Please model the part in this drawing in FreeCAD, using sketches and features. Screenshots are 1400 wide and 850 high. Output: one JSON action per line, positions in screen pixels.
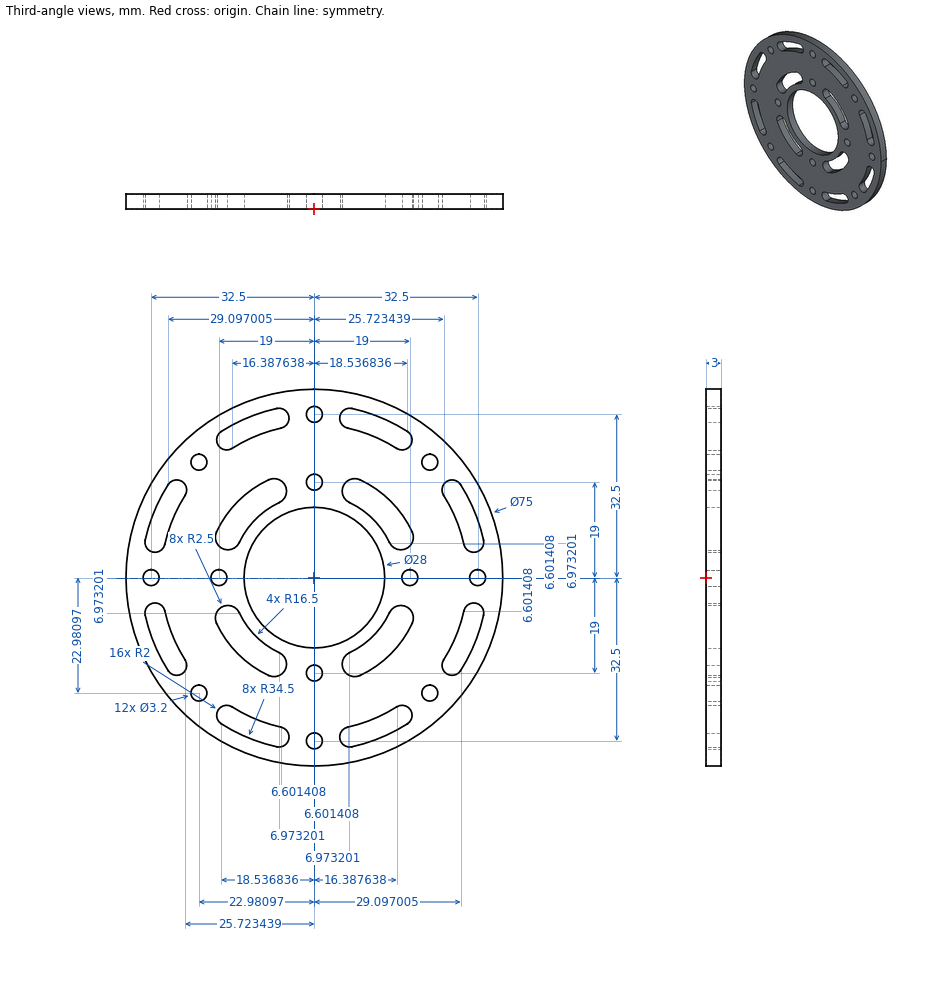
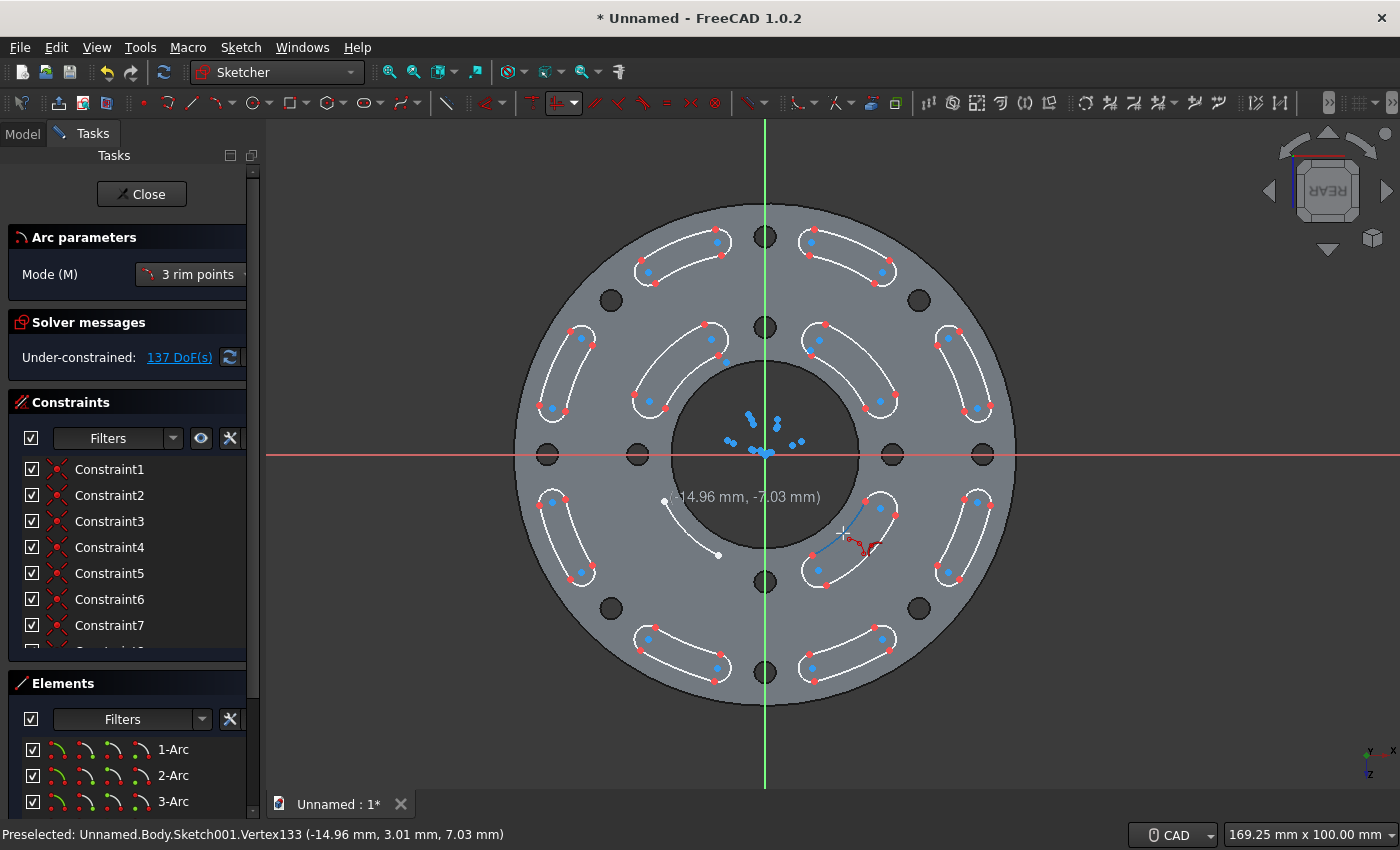
{"action": "left_click", "coordinate": [635, 516]}
{"action": "left_click", "coordinate": [643, 493]}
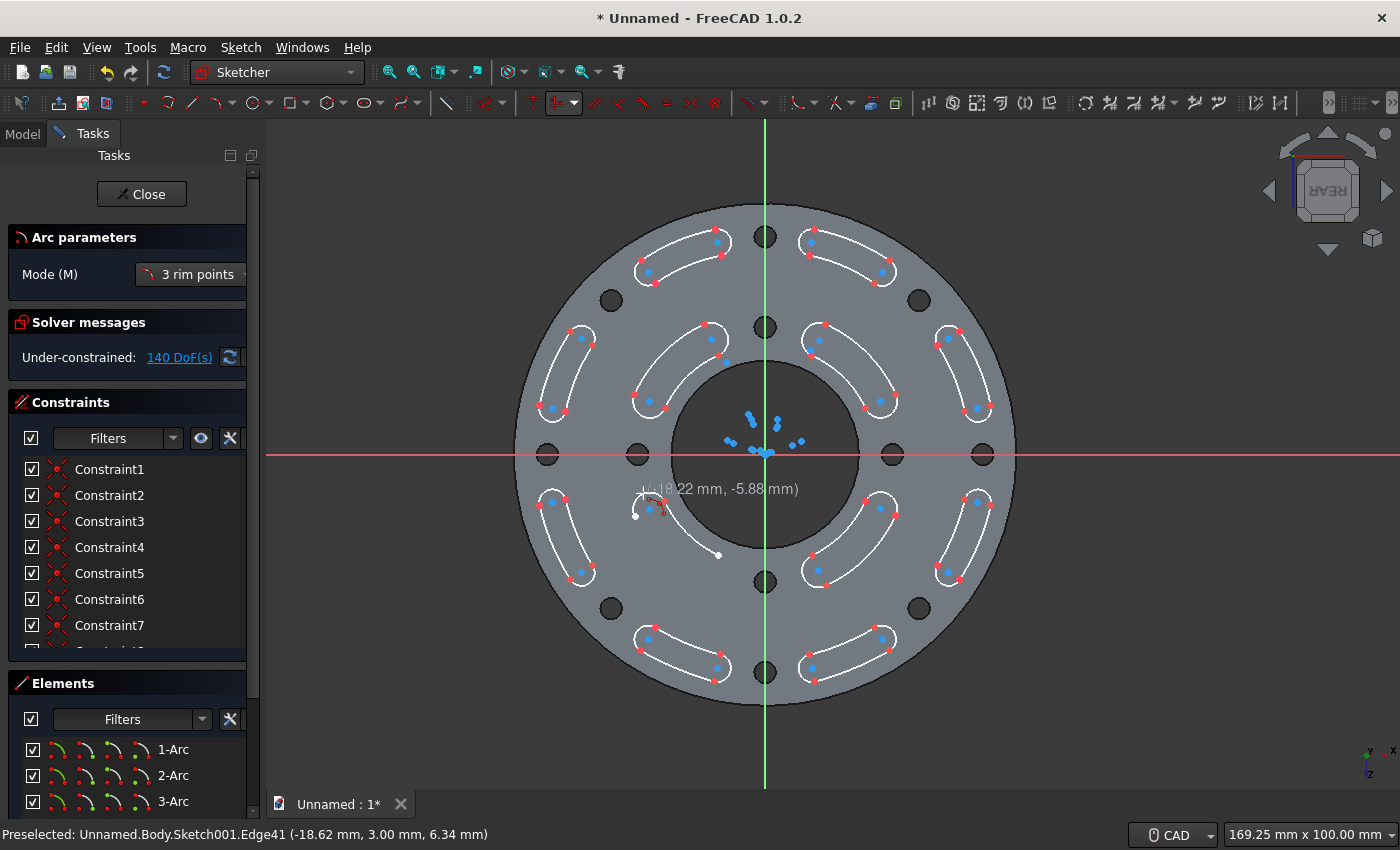
{"action": "left_click", "coordinate": [635, 517]}
{"action": "left_click", "coordinate": [704, 585]}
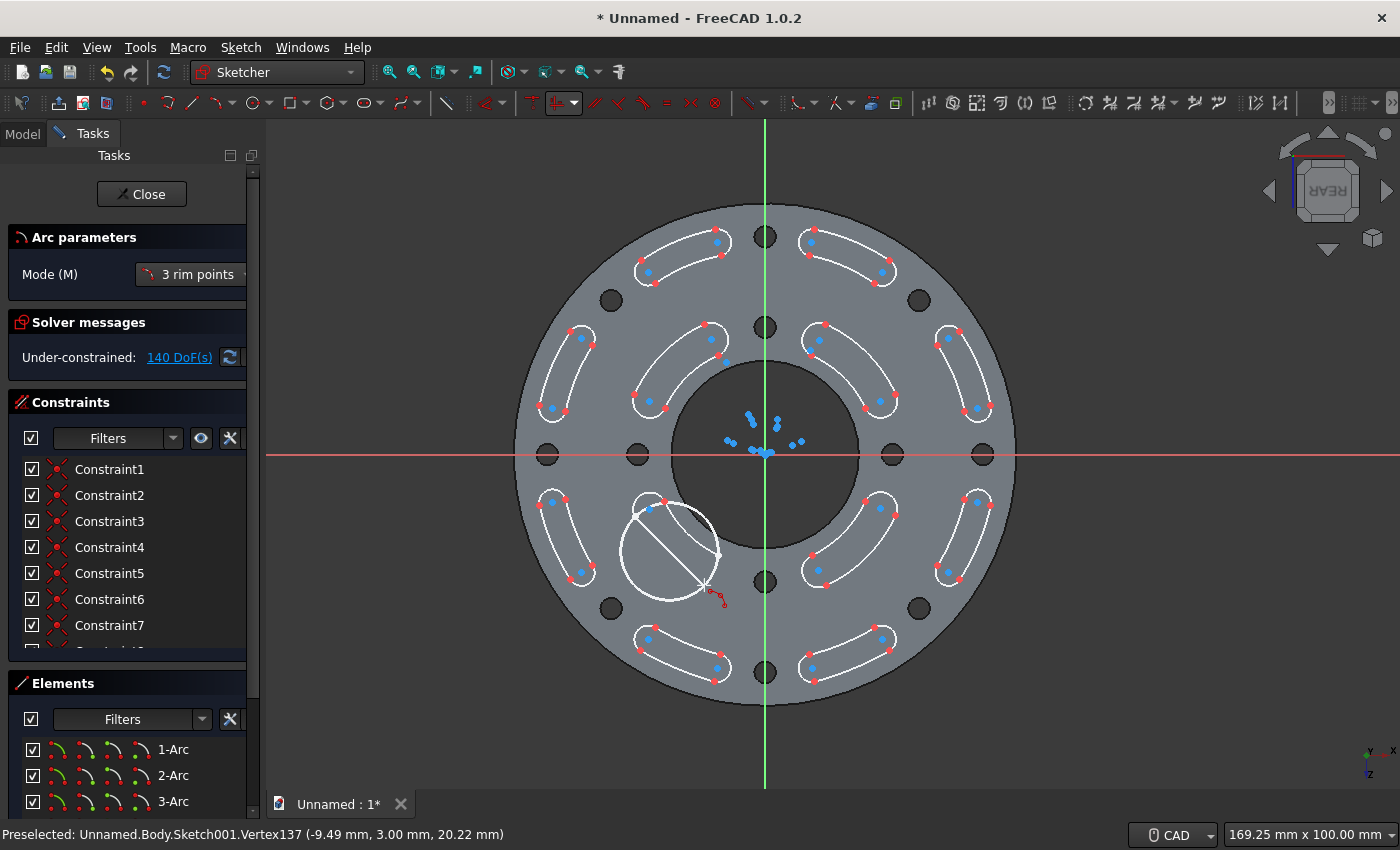
{"action": "scroll", "coordinate": [663, 556], "scroll_direction": "up", "scroll_amount": 4}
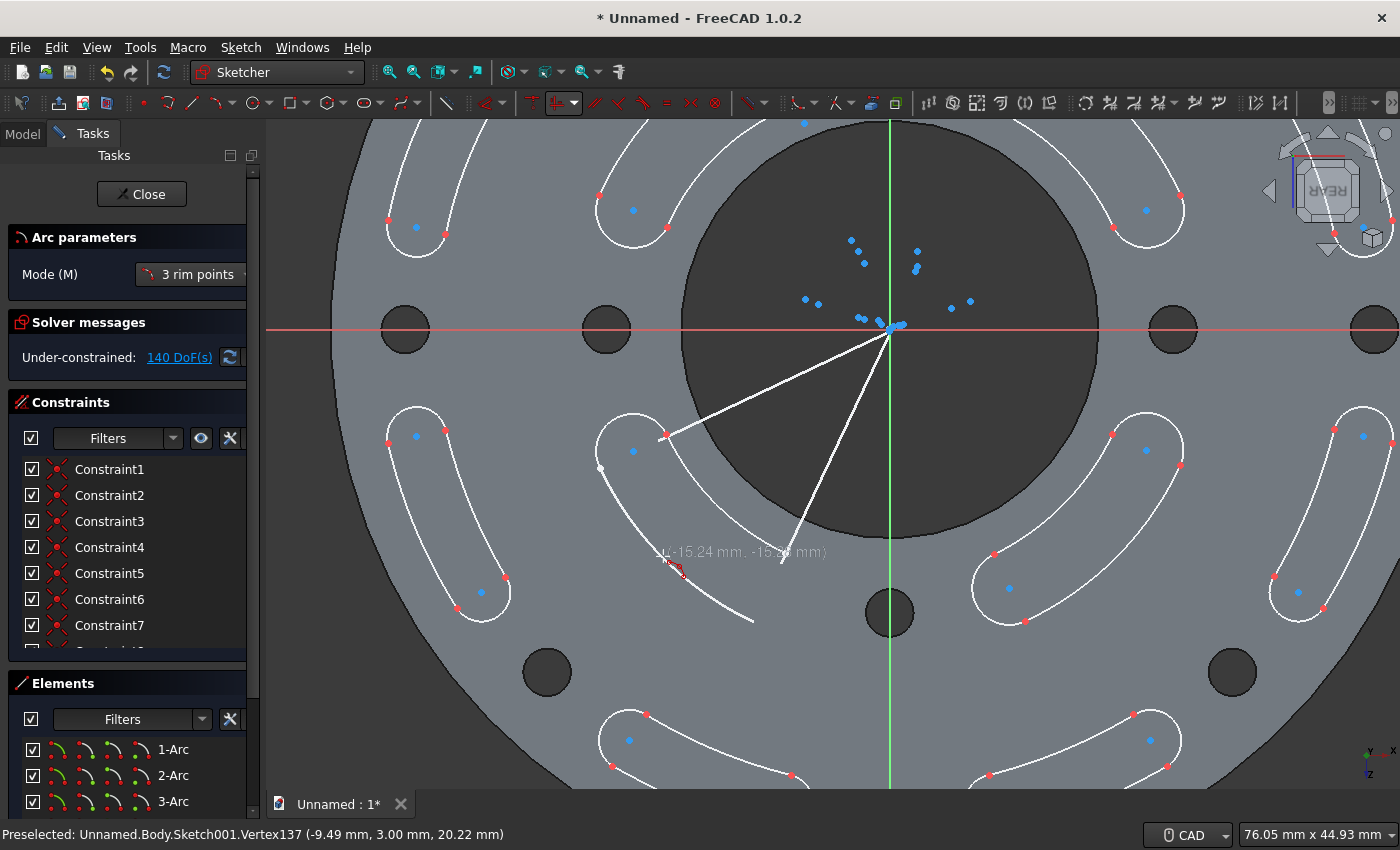
{"action": "left_click", "coordinate": [663, 556]}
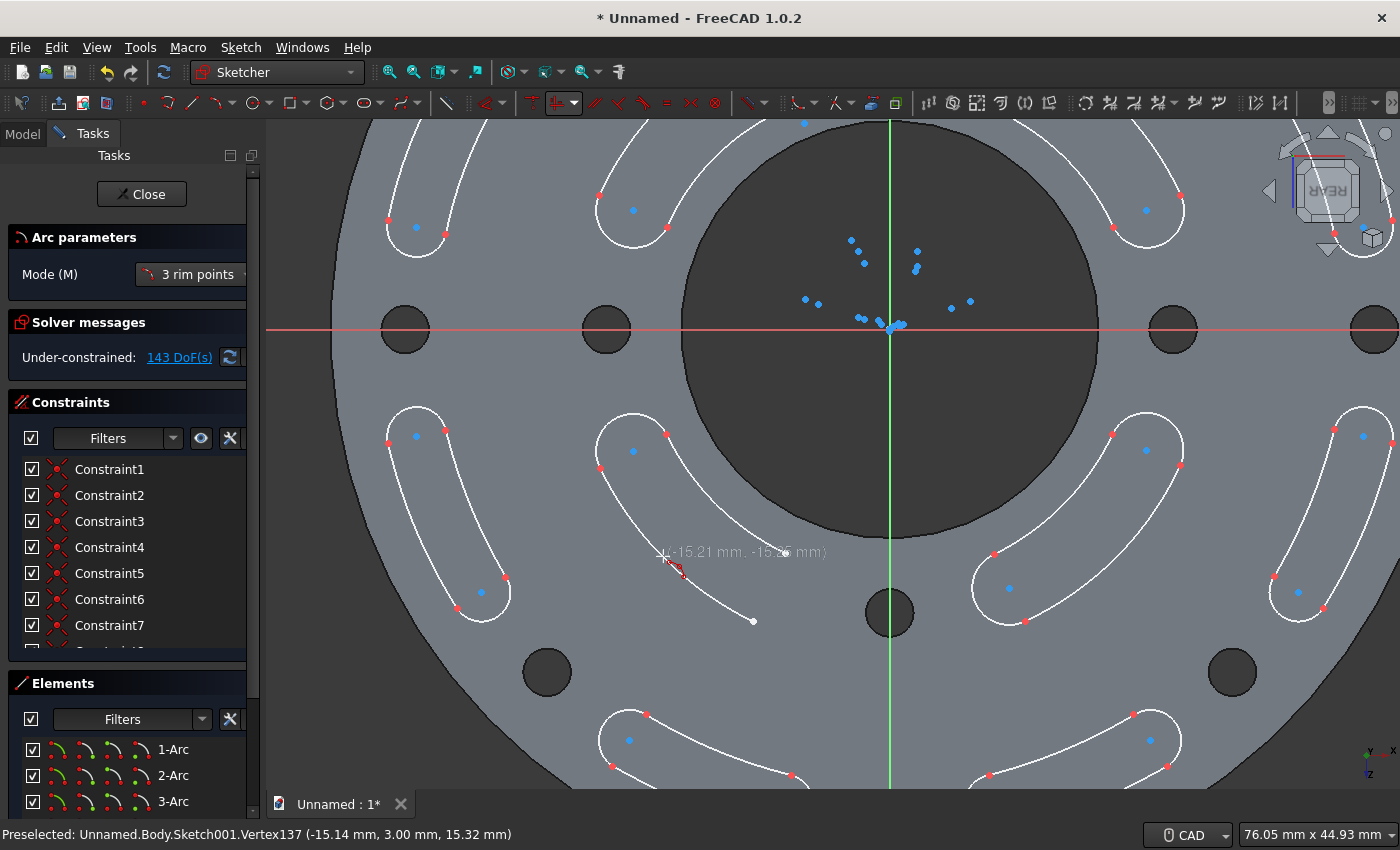
{"action": "left_click", "coordinate": [754, 622]}
{"action": "left_click", "coordinate": [786, 553]}
{"action": "left_click", "coordinate": [804, 602]}
{"action": "key", "text": "Escape"}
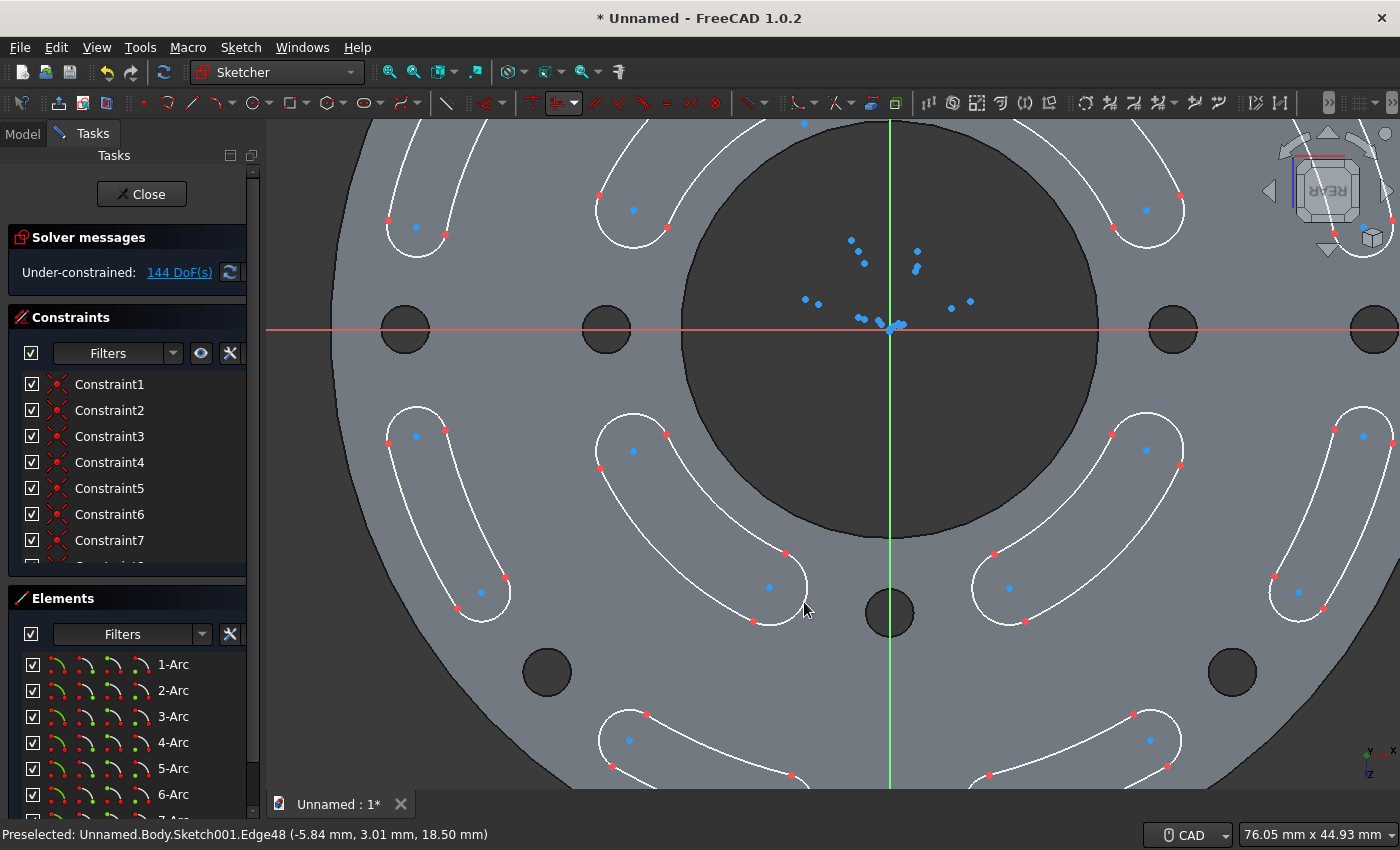
{"action": "scroll", "coordinate": [662, 556], "scroll_direction": "down", "scroll_amount": 4}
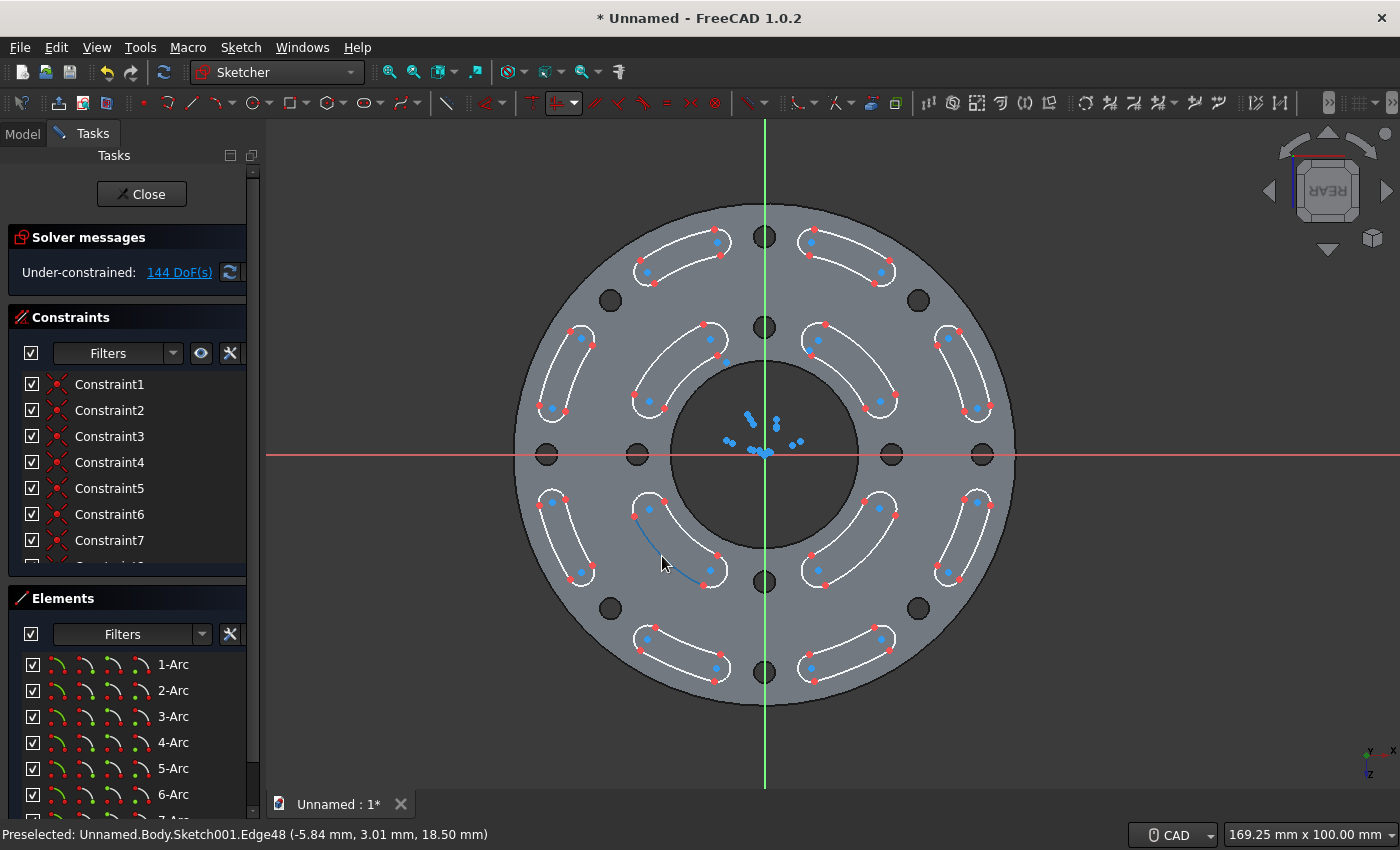
{"action": "left_click", "coordinate": [730, 248]}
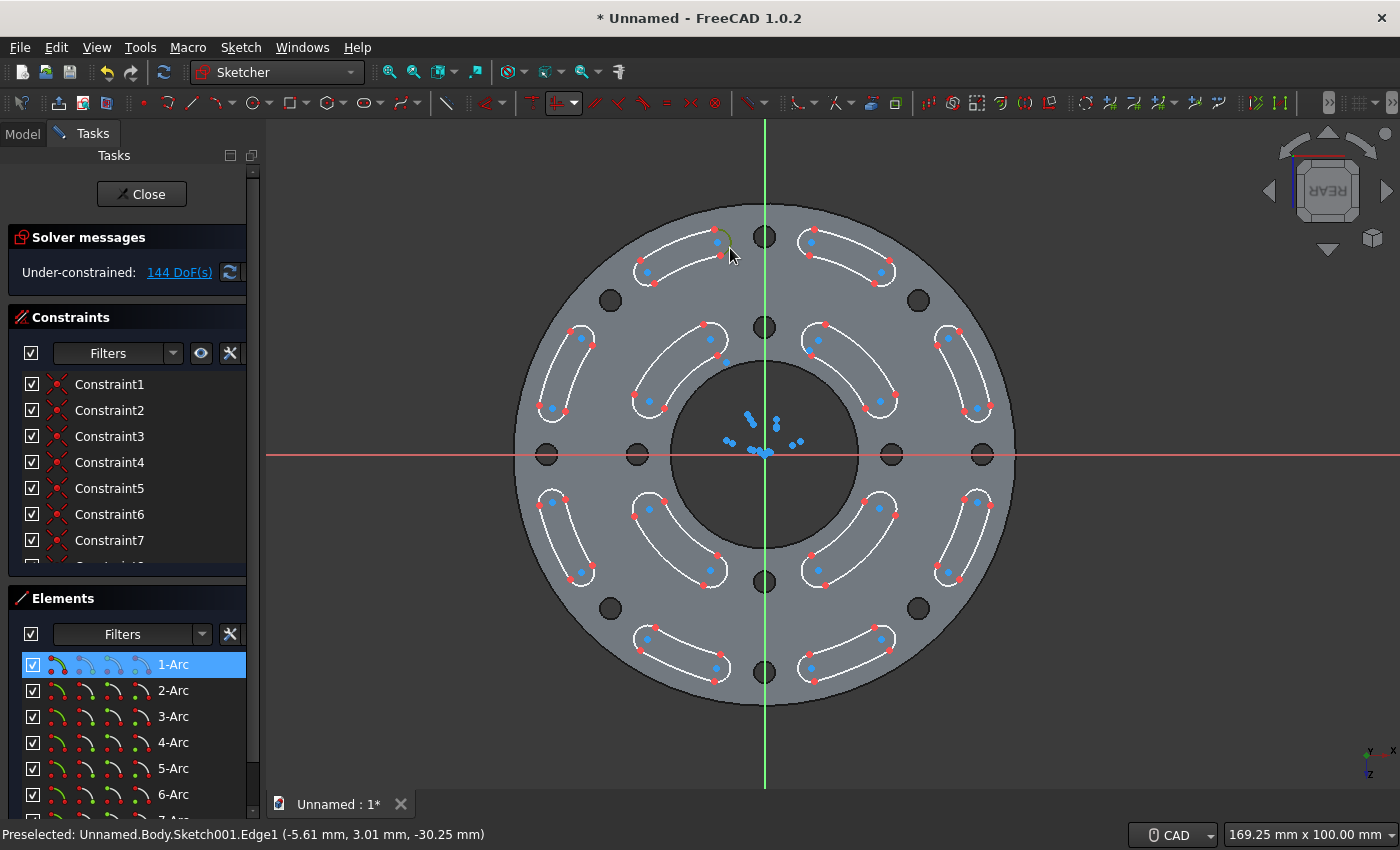
{"action": "left_click", "coordinate": [691, 236]}